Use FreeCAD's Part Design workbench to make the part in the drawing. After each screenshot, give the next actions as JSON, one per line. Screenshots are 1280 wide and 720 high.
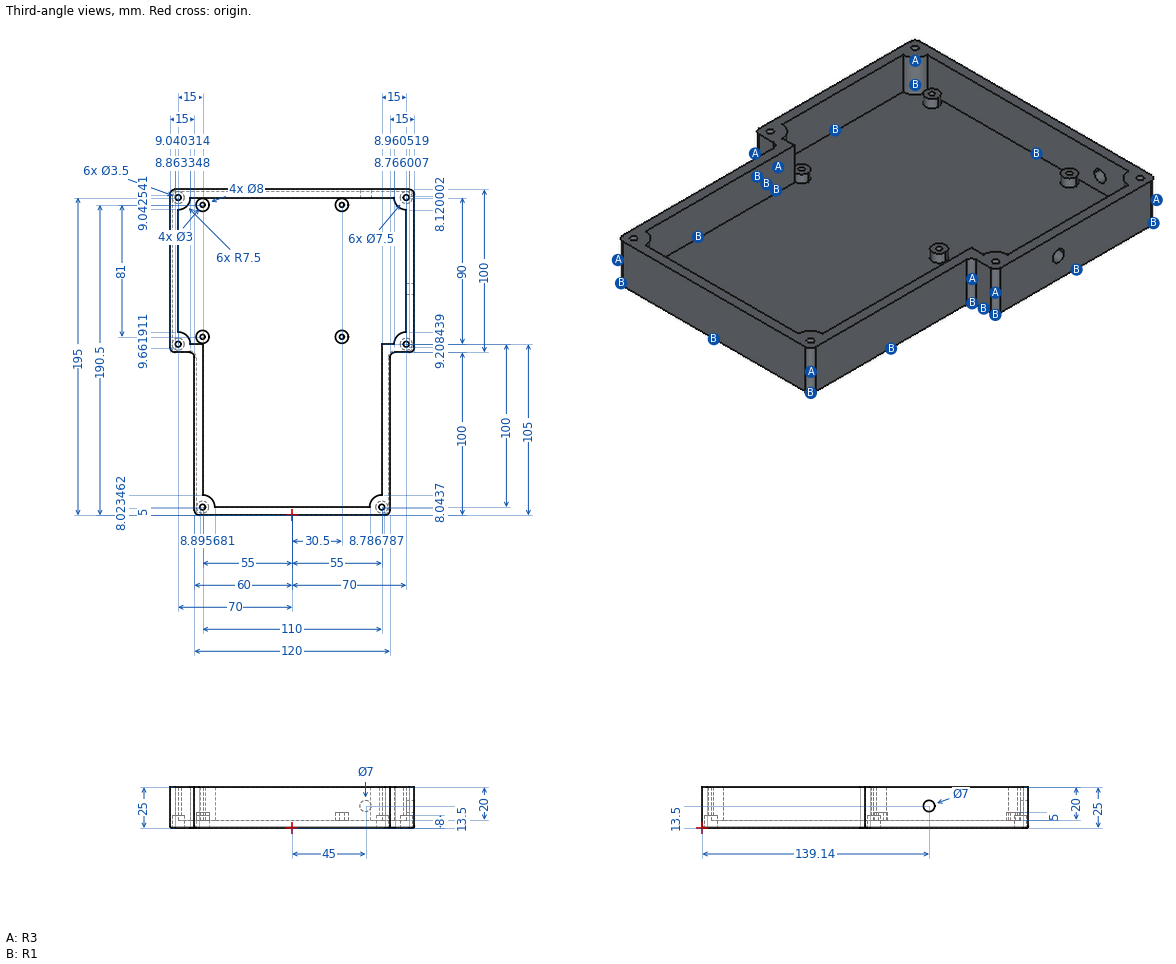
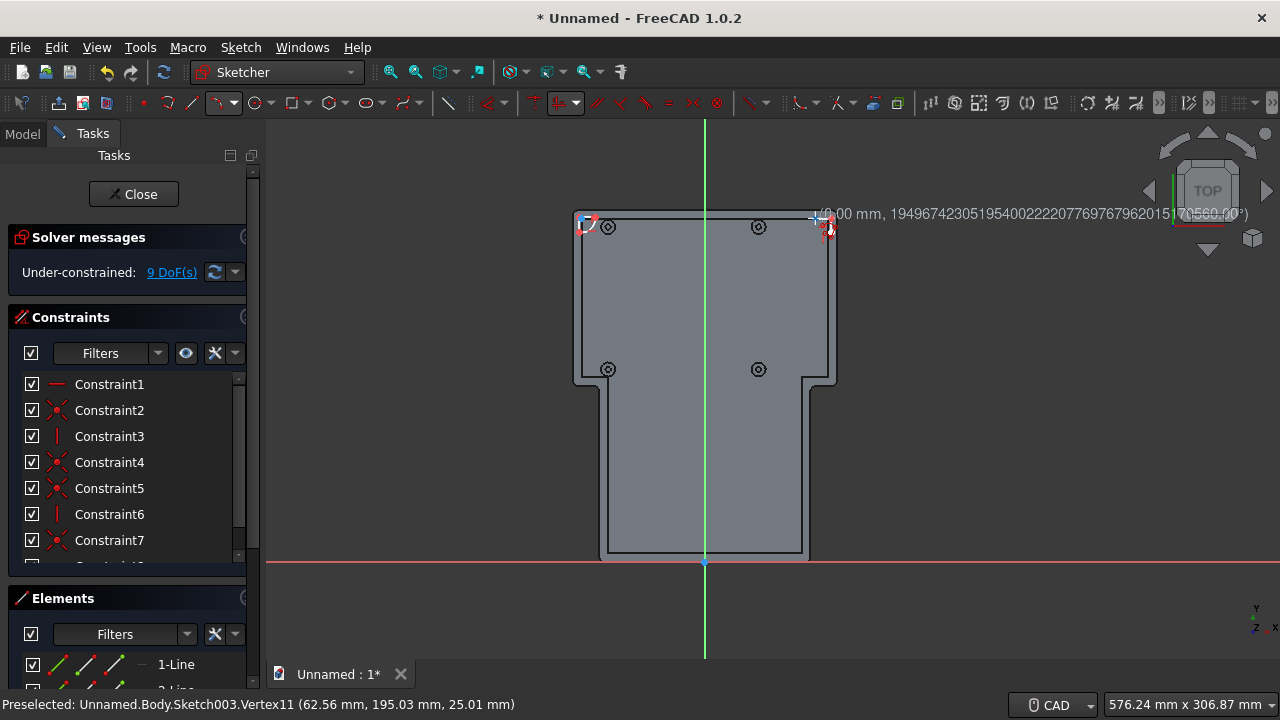
{"action": "left_click", "coordinate": [218, 104]}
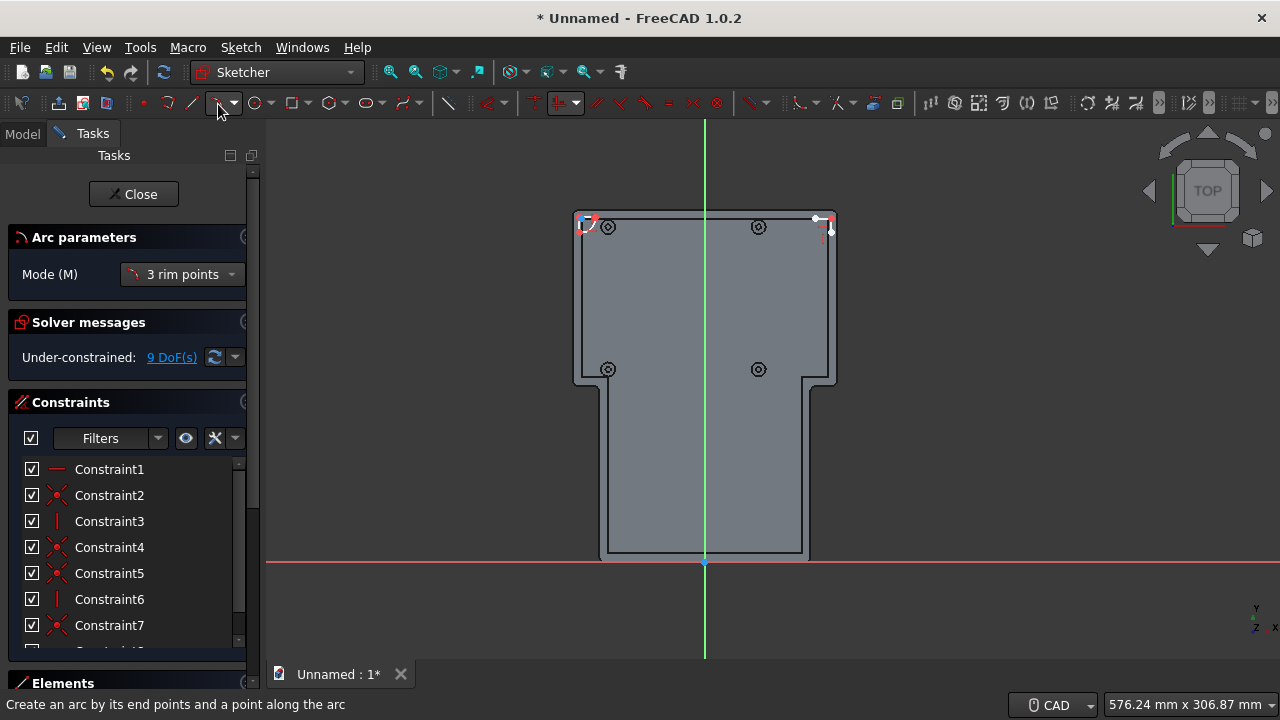
{"action": "scroll", "coordinate": [815, 218], "scroll_direction": "up", "scroll_amount": 4}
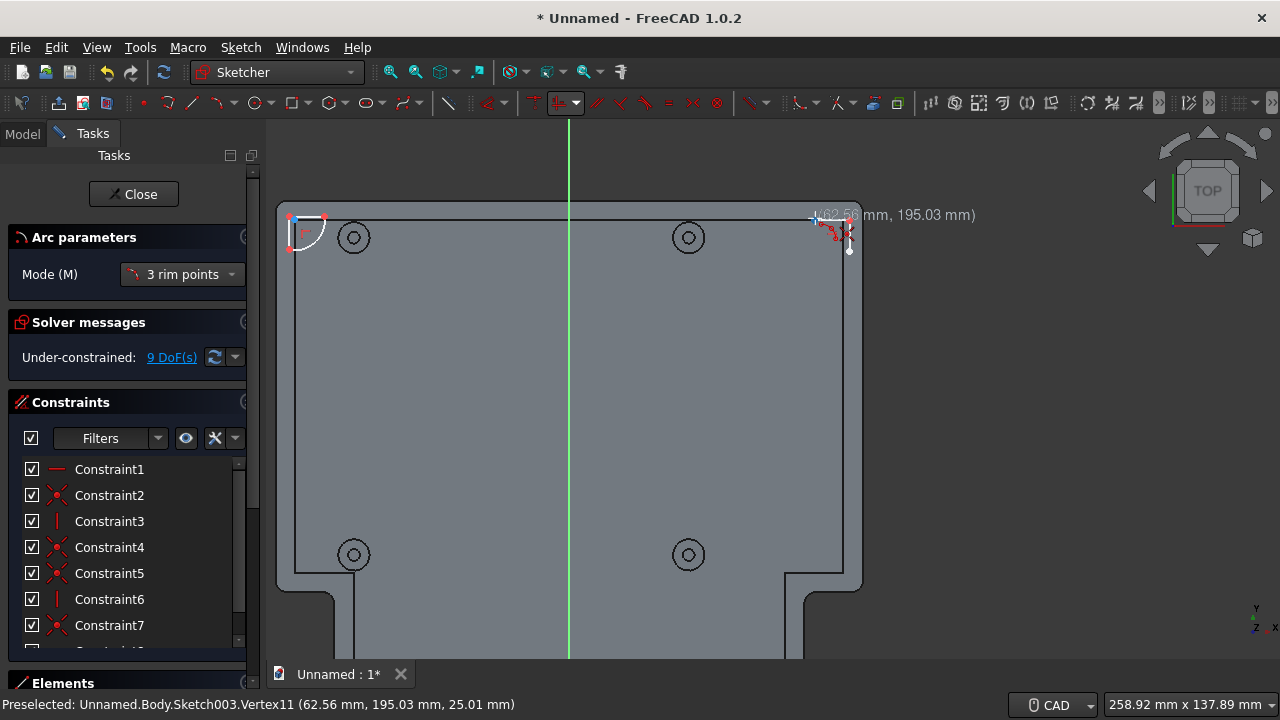
{"action": "left_click", "coordinate": [814, 220]}
{"action": "left_click", "coordinate": [850, 251]}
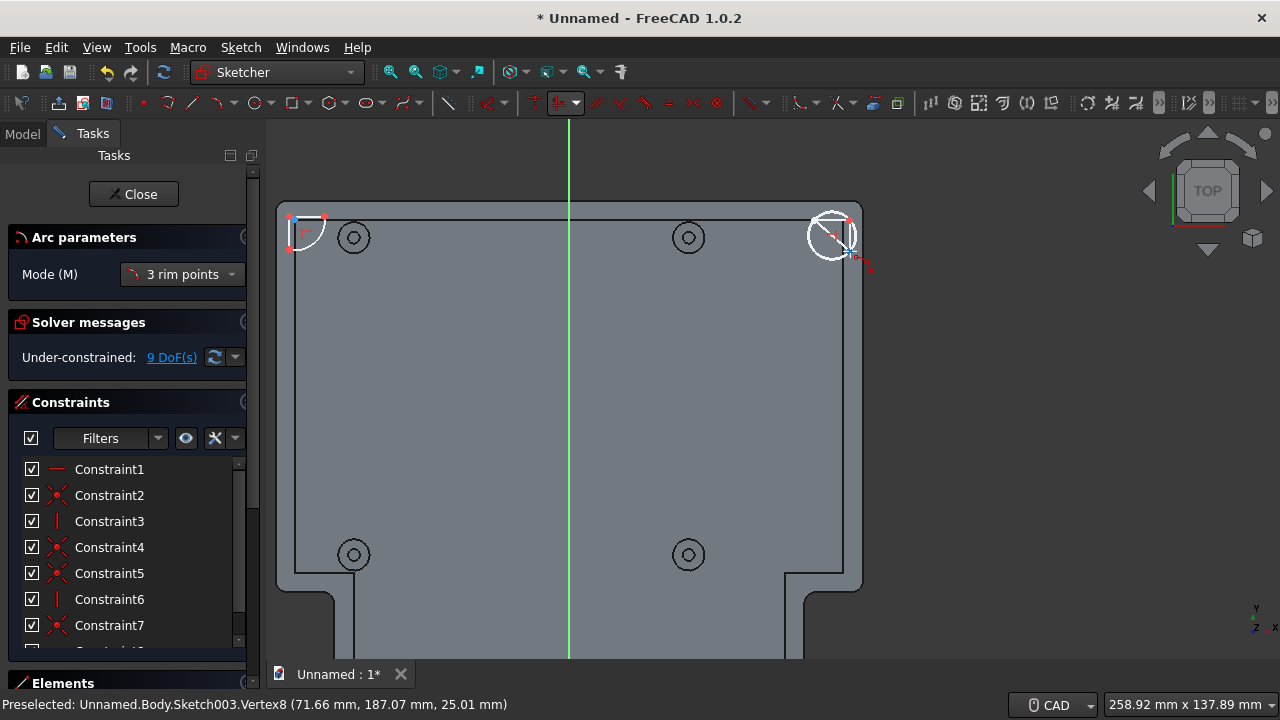
{"action": "scroll", "coordinate": [824, 242], "scroll_direction": "up", "scroll_amount": 2}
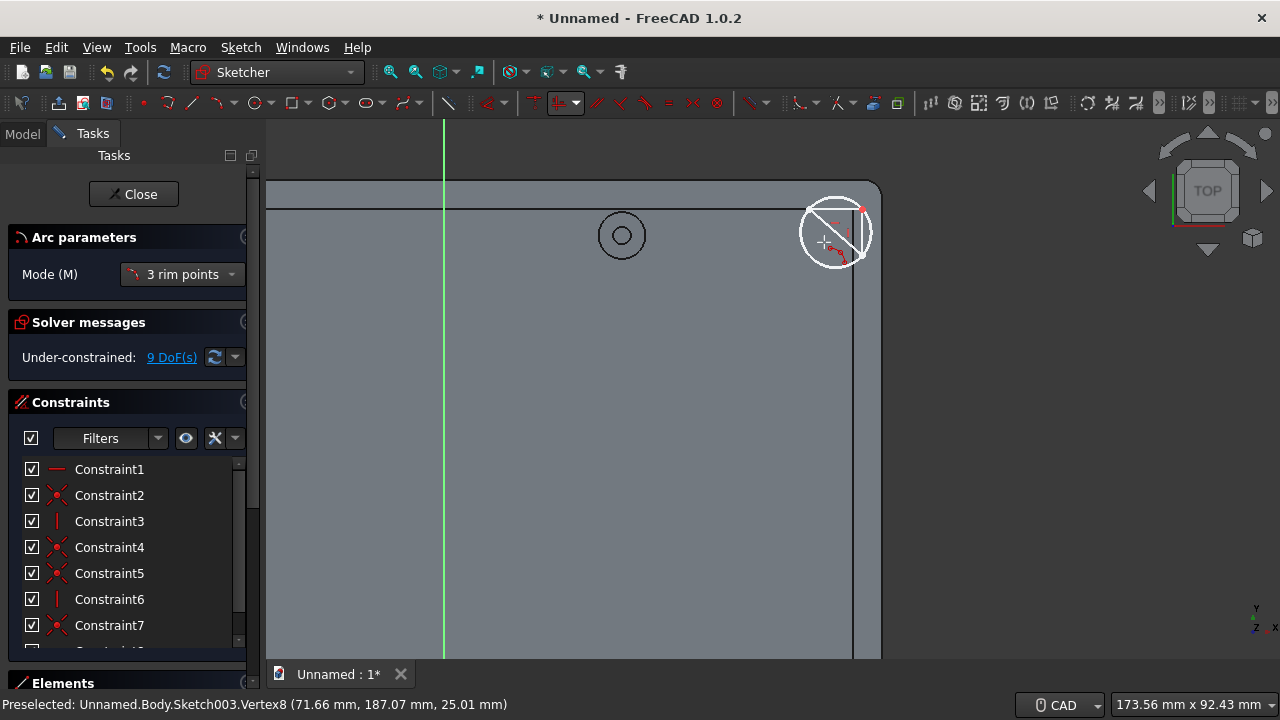
{"action": "left_click", "coordinate": [823, 242]}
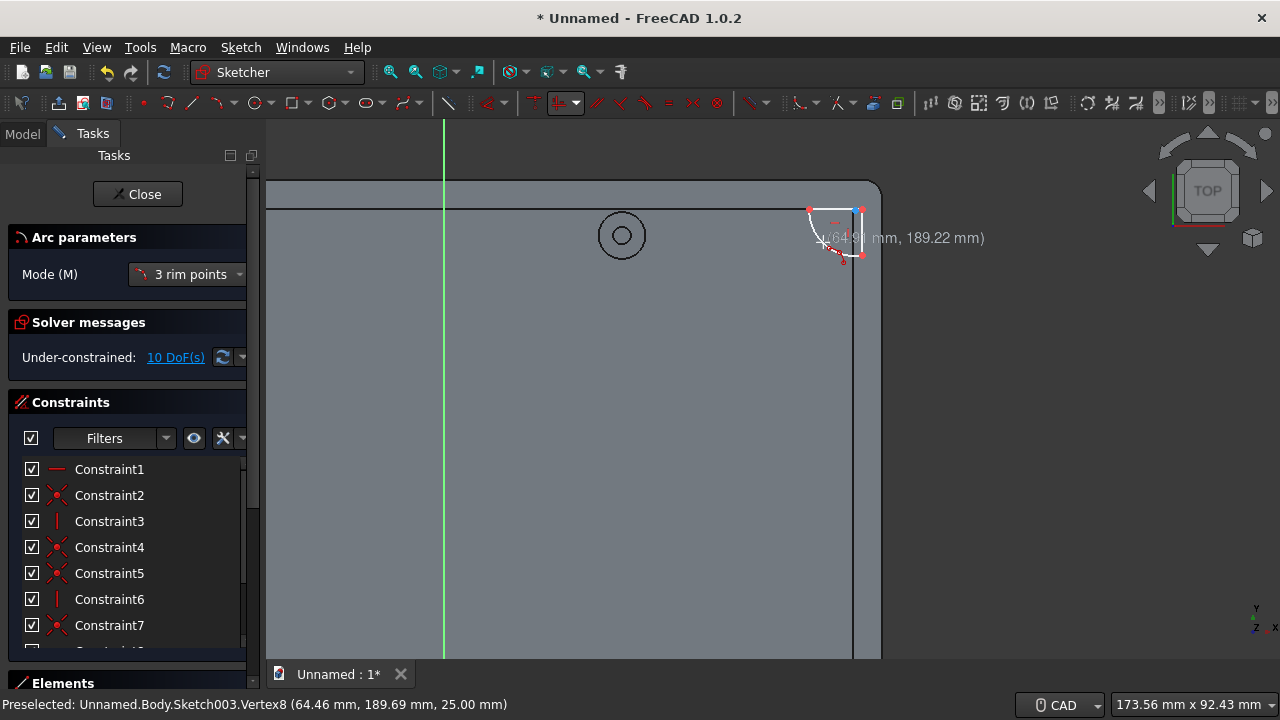
{"action": "key", "text": "g m"}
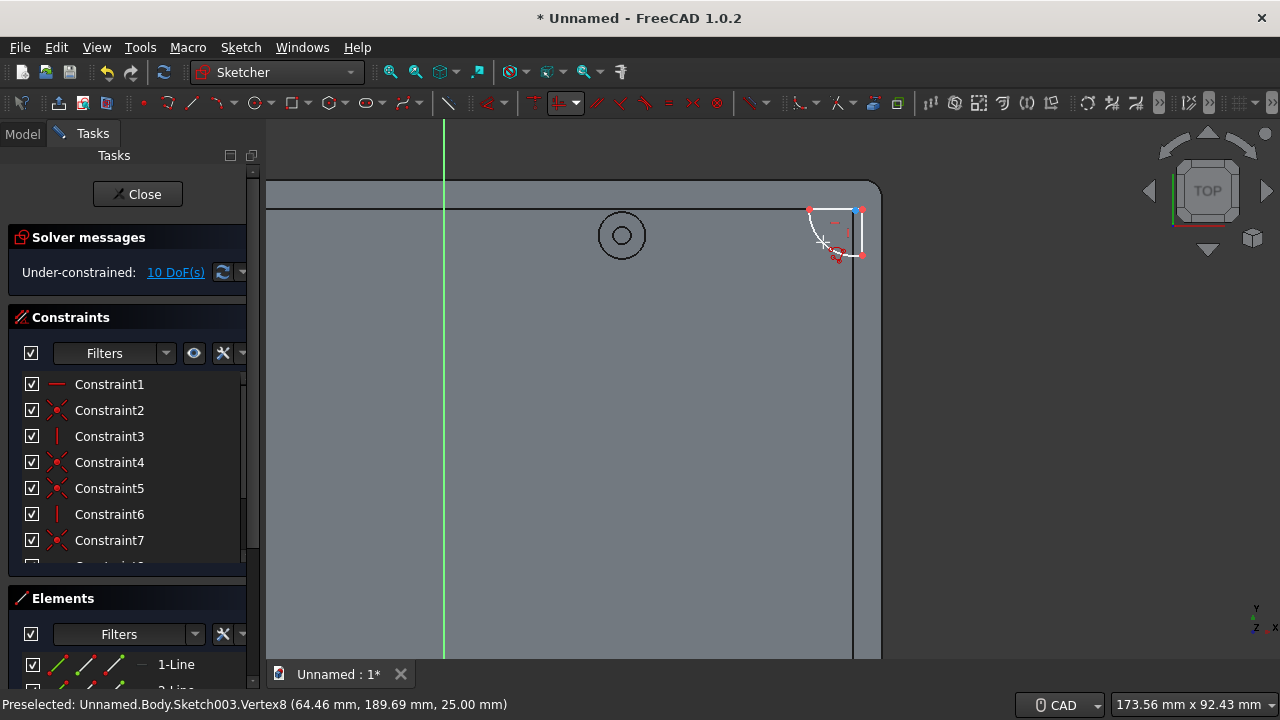
{"action": "scroll", "coordinate": [817, 223], "scroll_direction": "down", "scroll_amount": 6}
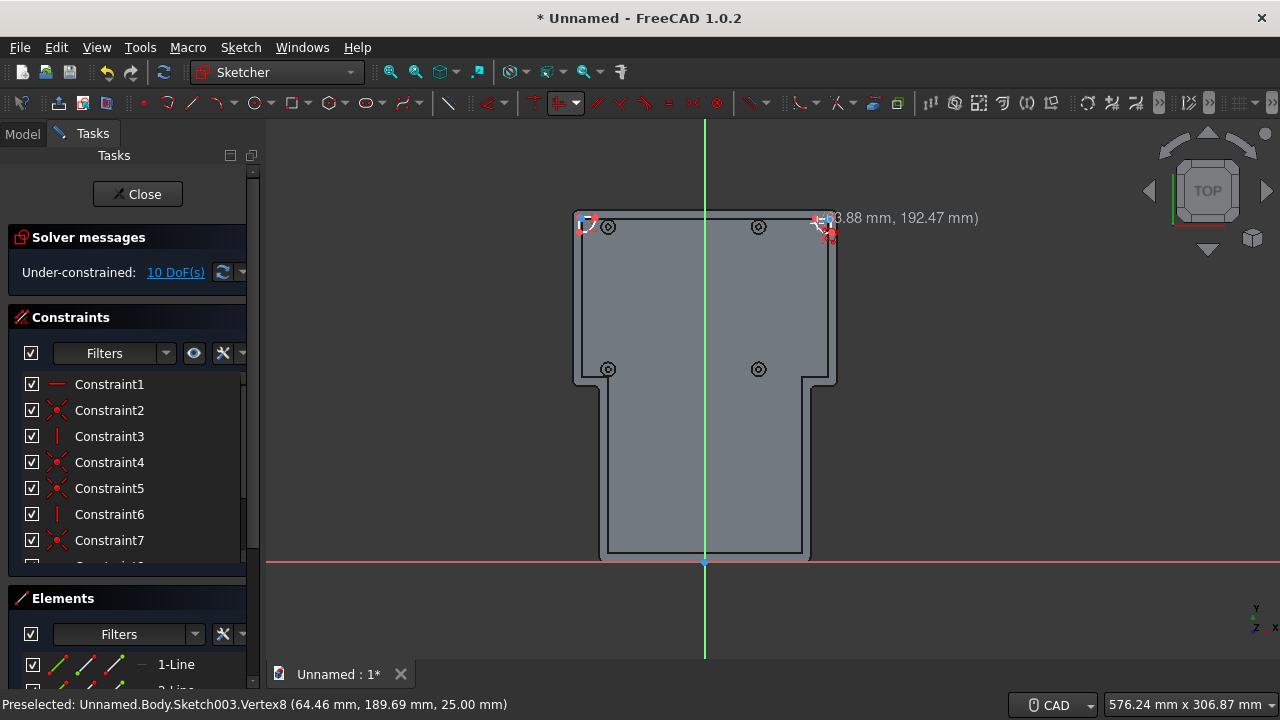
{"action": "left_click", "coordinate": [815, 381]}
{"action": "left_click", "coordinate": [831, 381]}
{"action": "left_click", "coordinate": [831, 364]}
{"action": "right_click", "coordinate": [831, 364]}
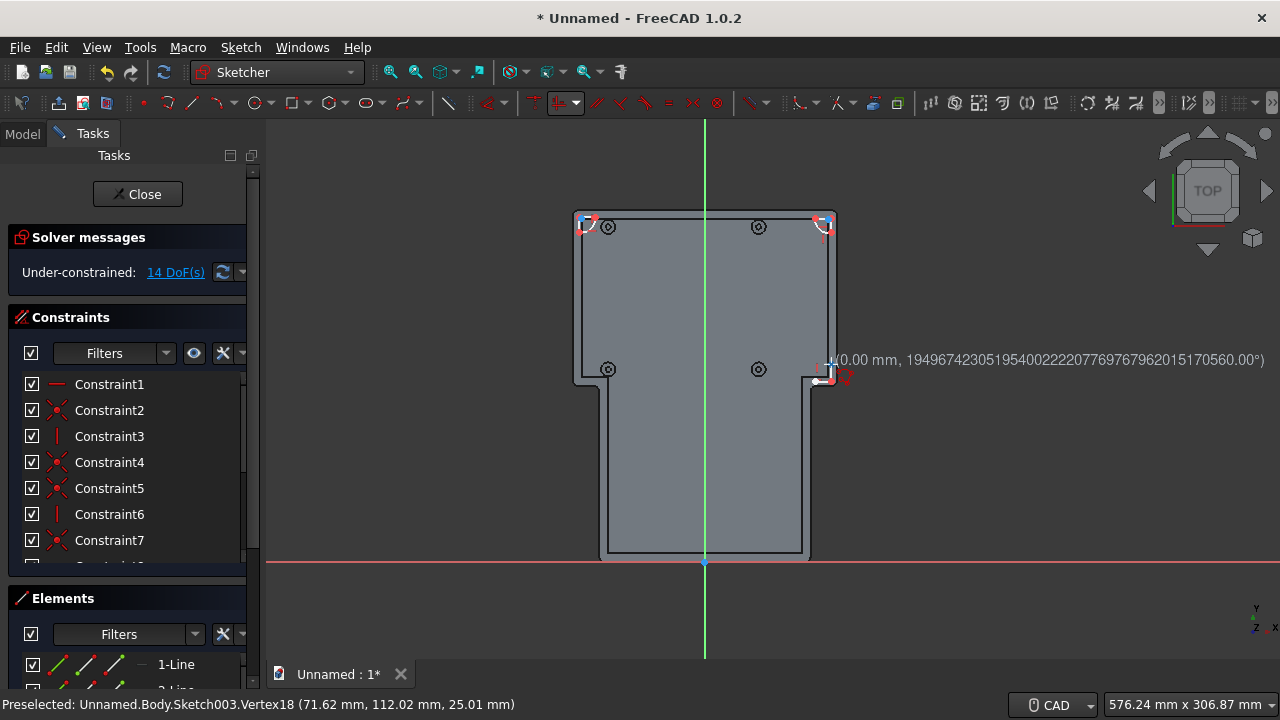
{"action": "key", "text": "g 3 a"}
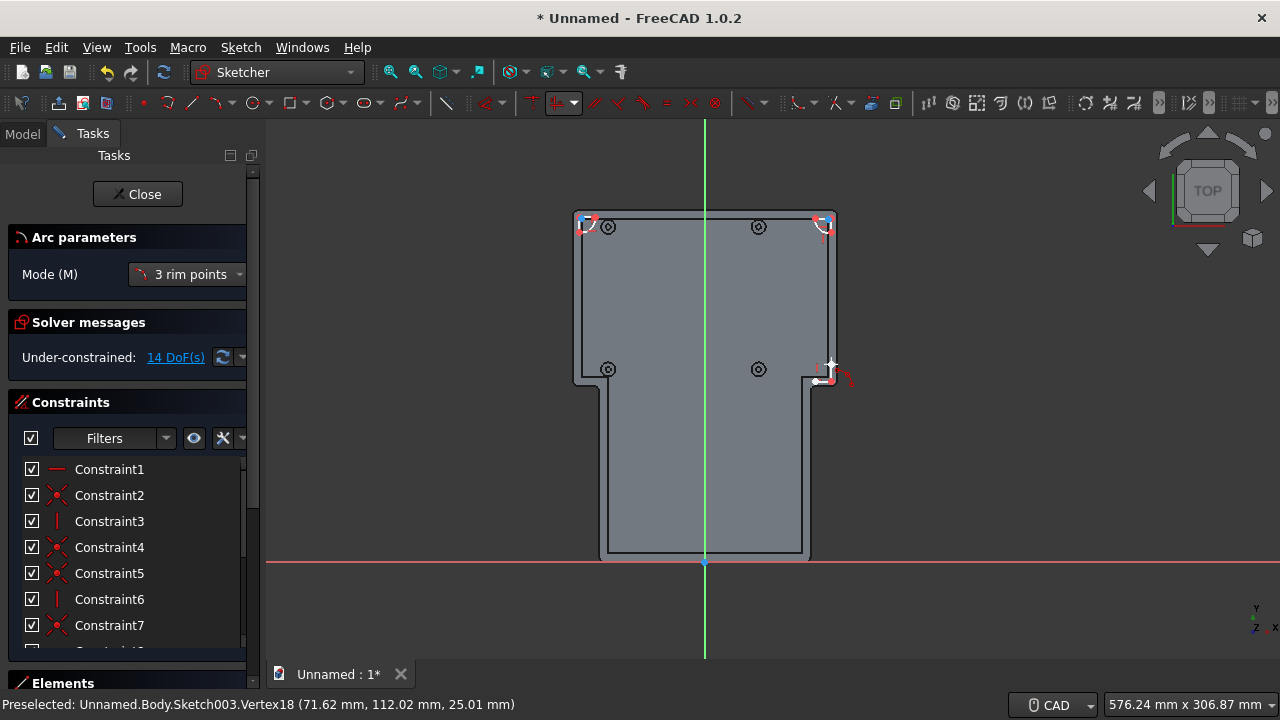
{"action": "scroll", "coordinate": [831, 364], "scroll_direction": "up", "scroll_amount": 4}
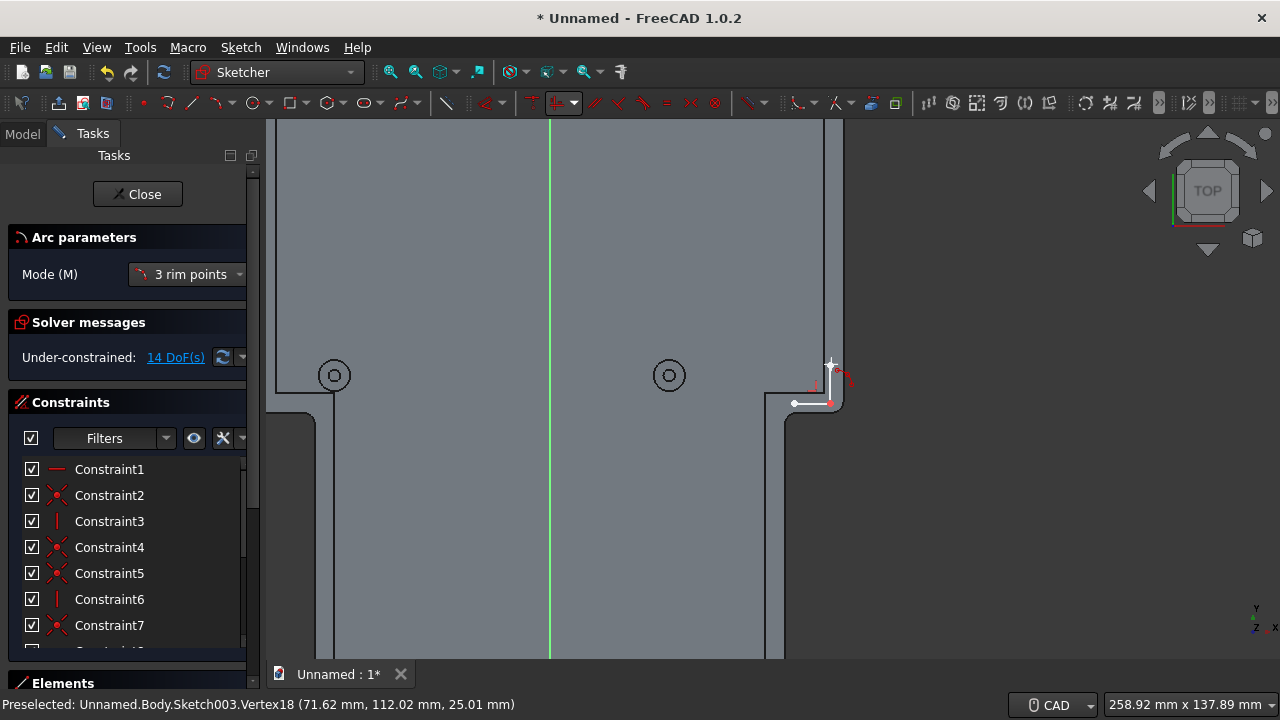
{"action": "left_click", "coordinate": [830, 366]}
{"action": "left_click", "coordinate": [795, 404]}
{"action": "left_click", "coordinate": [803, 373]}